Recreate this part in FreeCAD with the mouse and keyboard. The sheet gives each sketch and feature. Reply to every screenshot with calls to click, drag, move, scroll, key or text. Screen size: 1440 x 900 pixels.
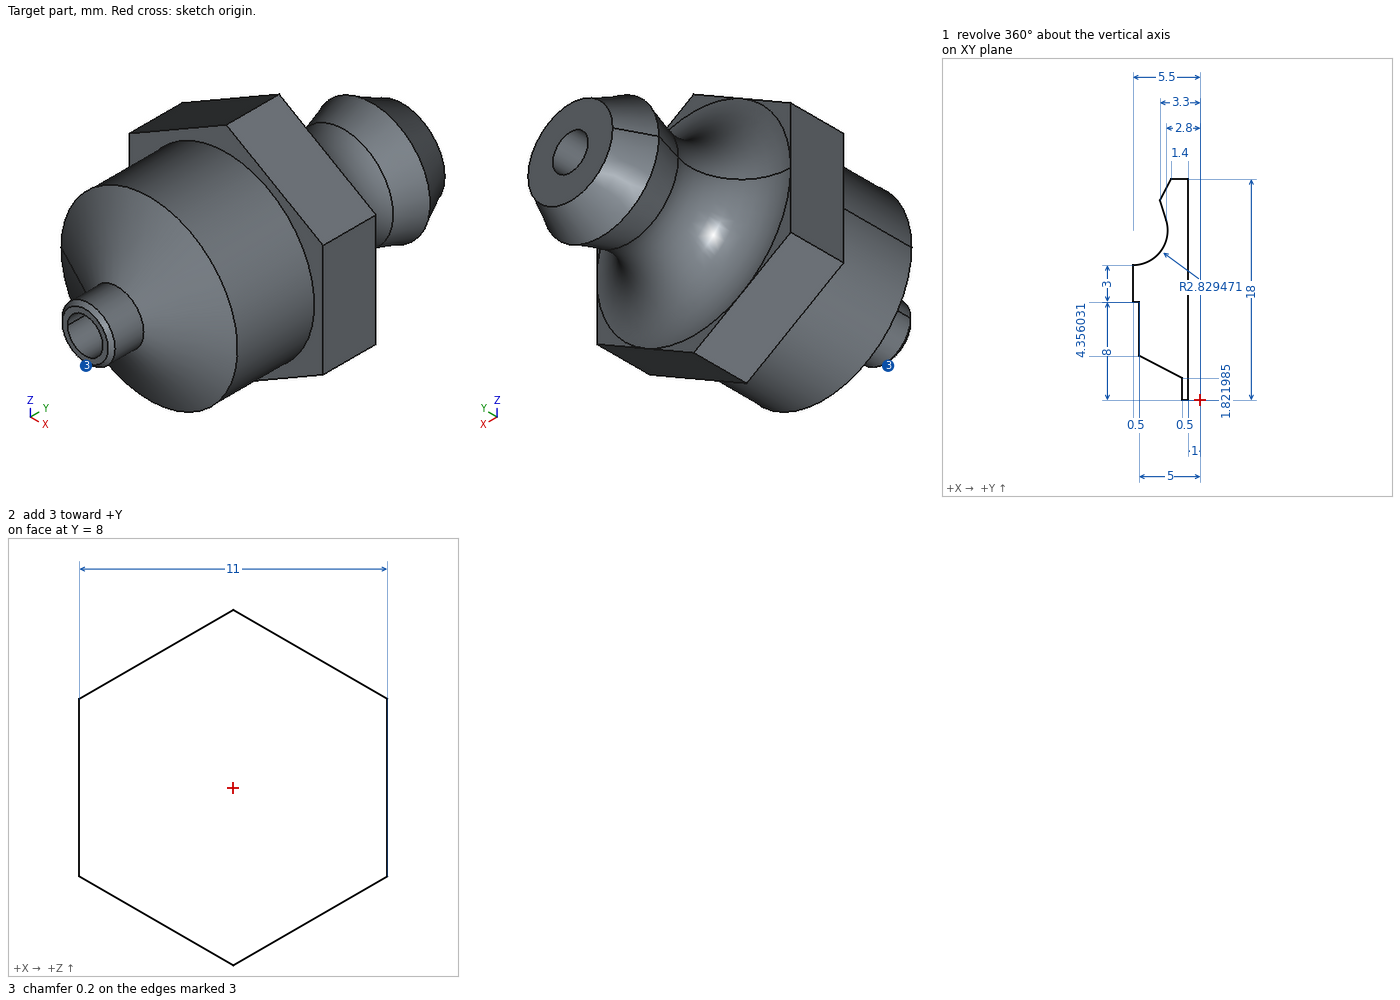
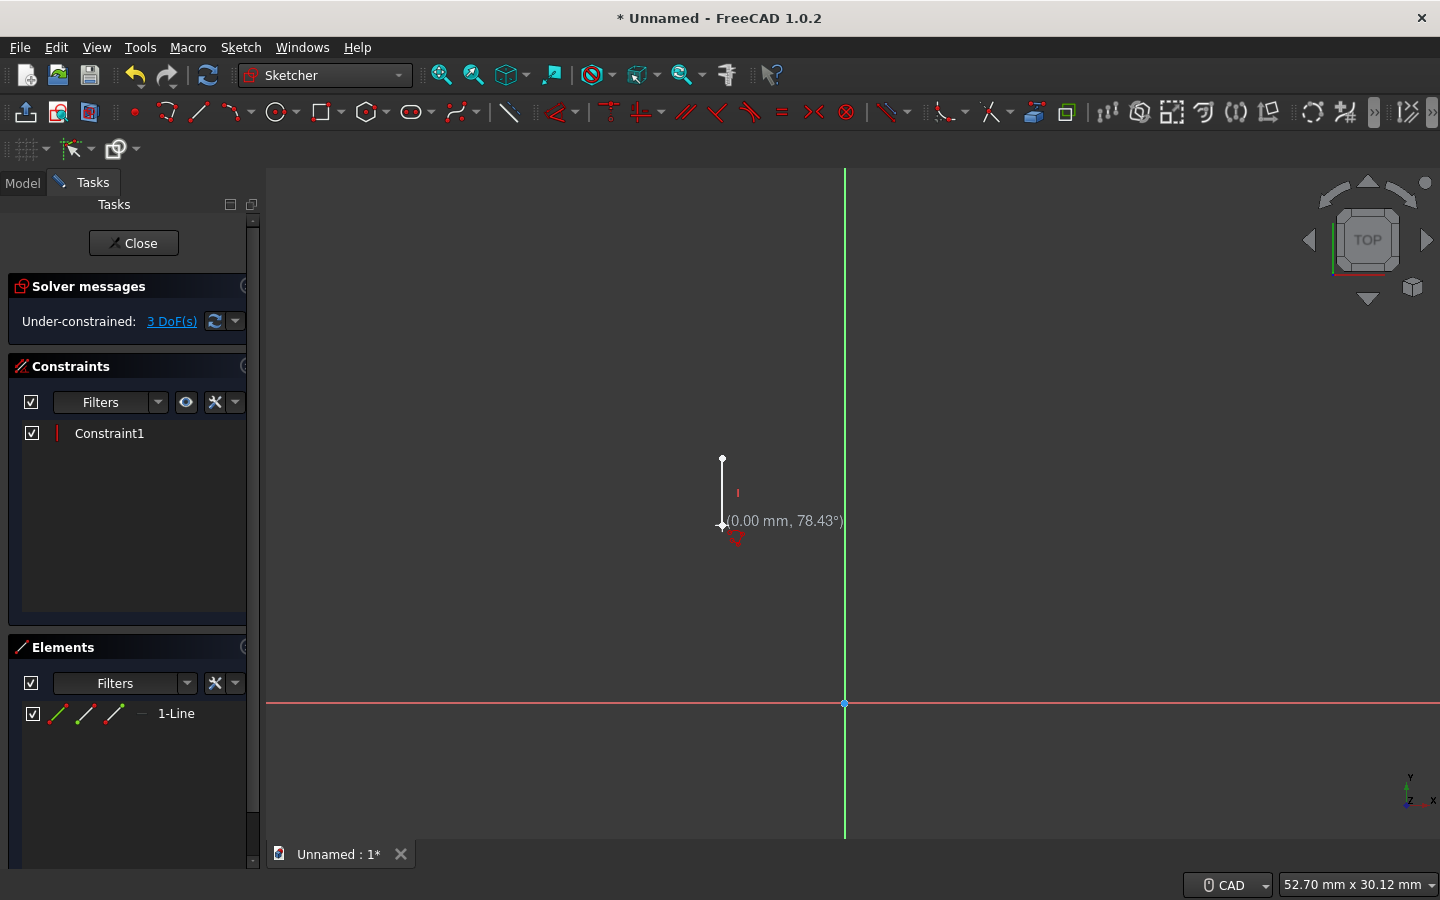
scroll(733, 525, up, 2)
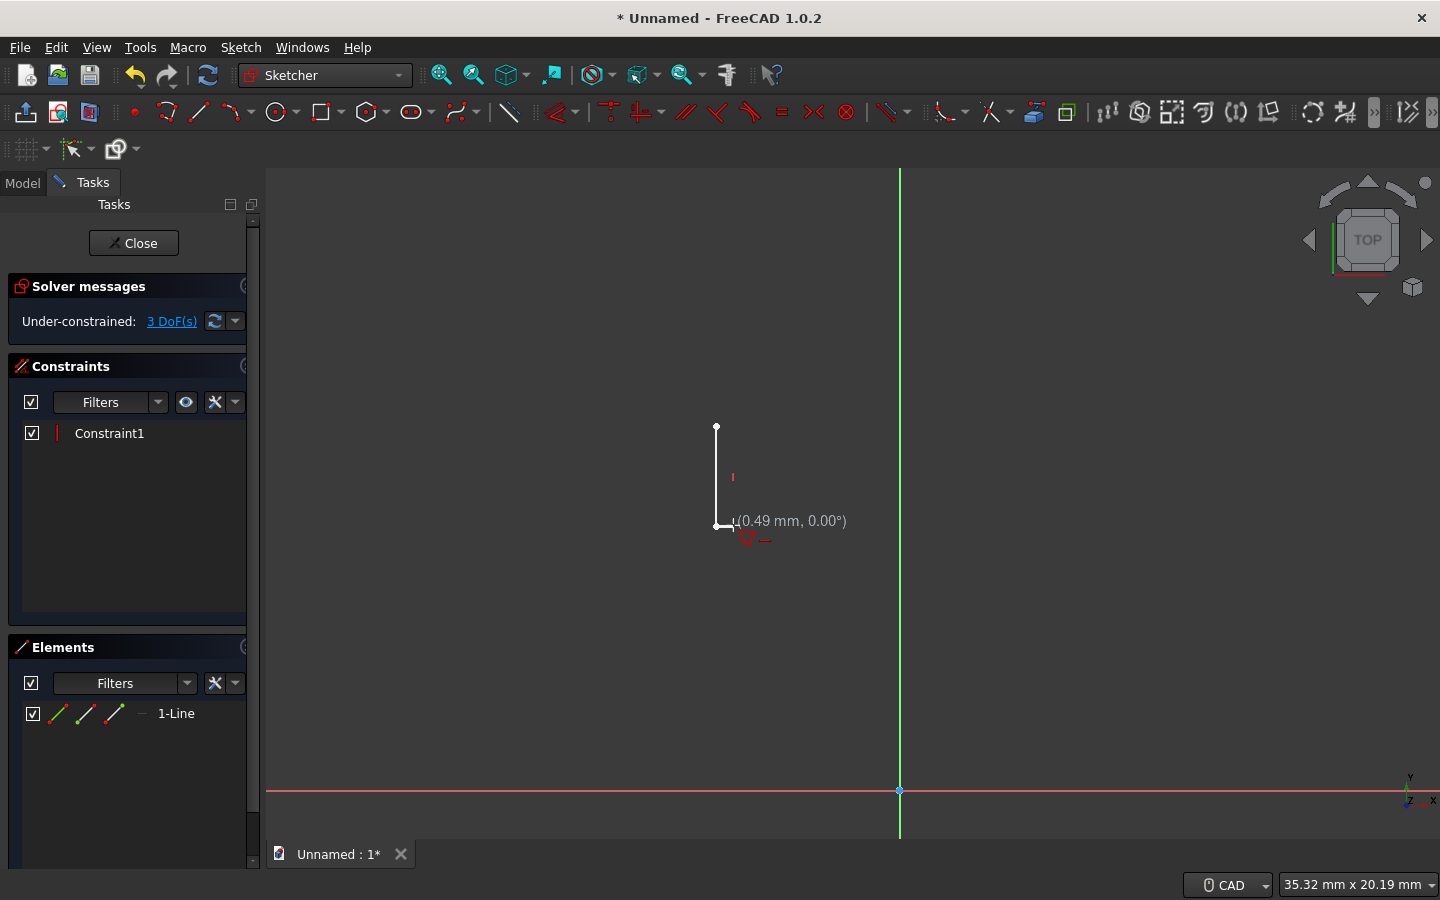
click(734, 525)
click(734, 670)
click(850, 730)
click(850, 791)
click(866, 782)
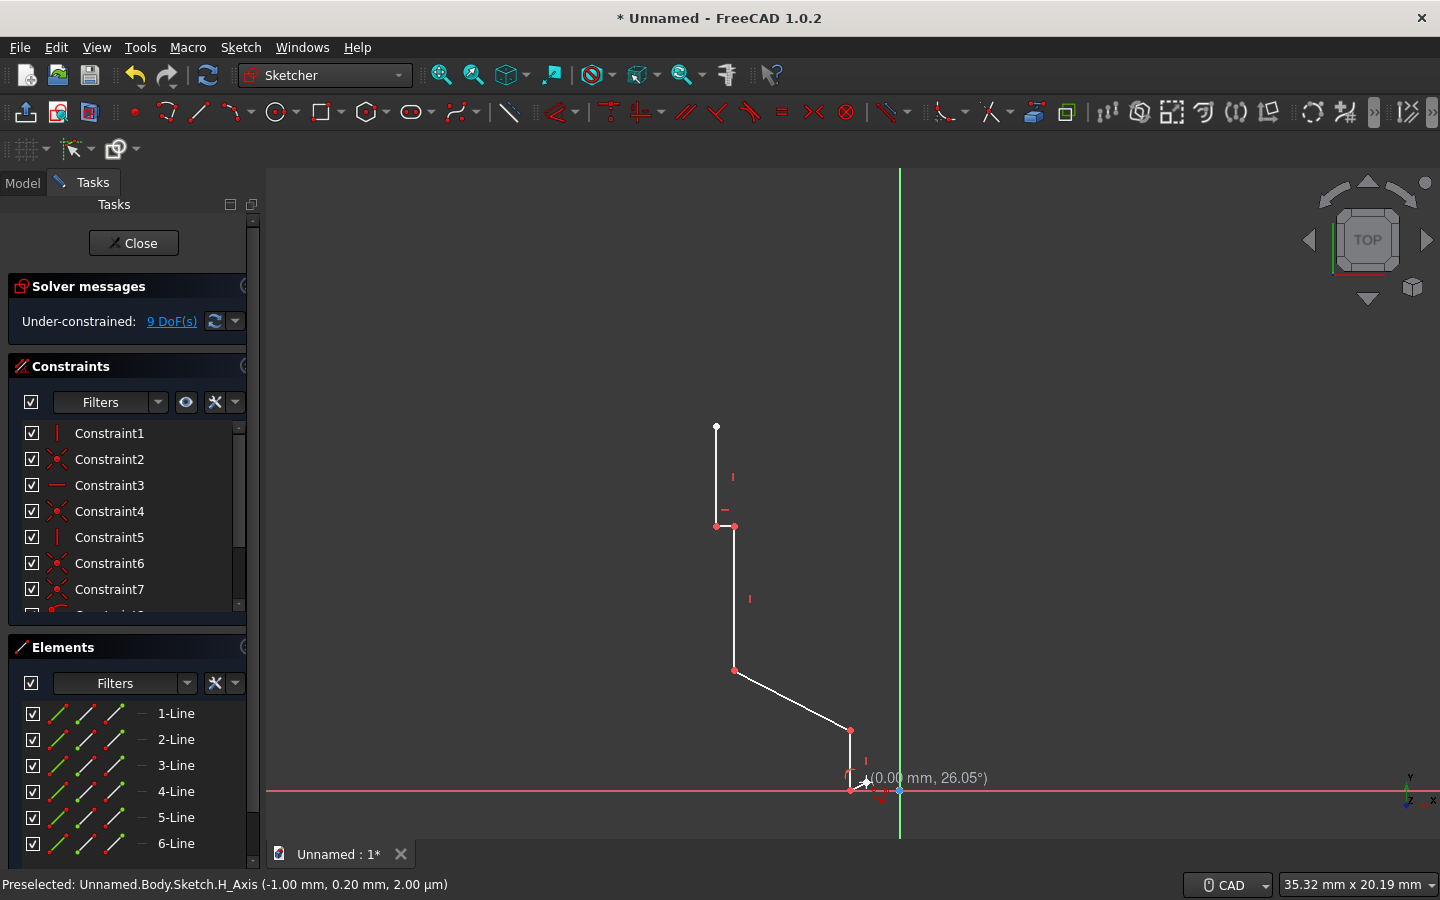
scroll(736, 528, down, 2)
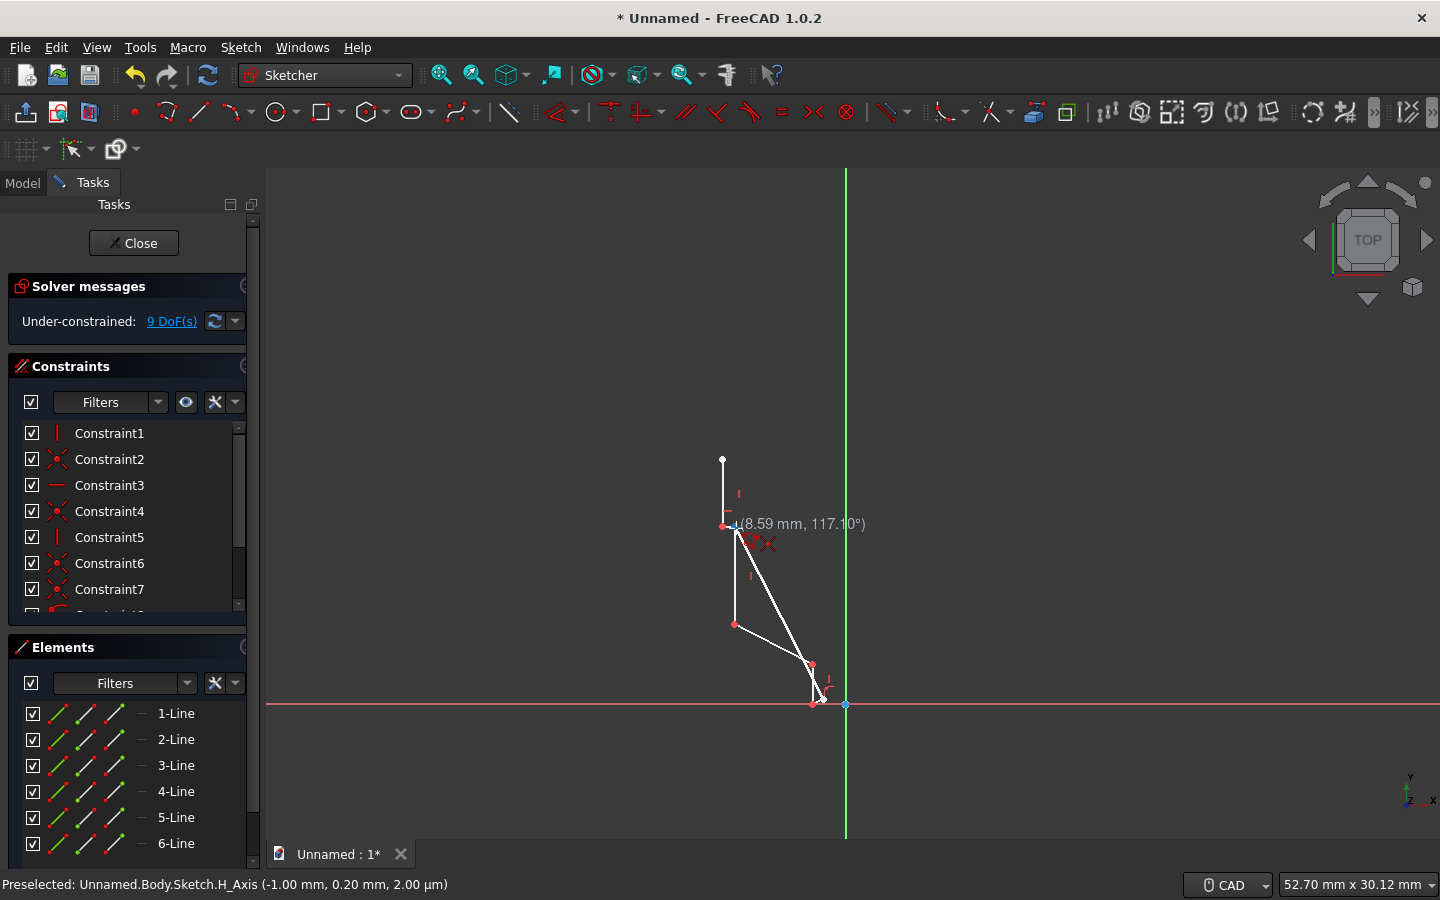
click(823, 303)
click(792, 303)
click(772, 342)
click(783, 377)
right_click(783, 377)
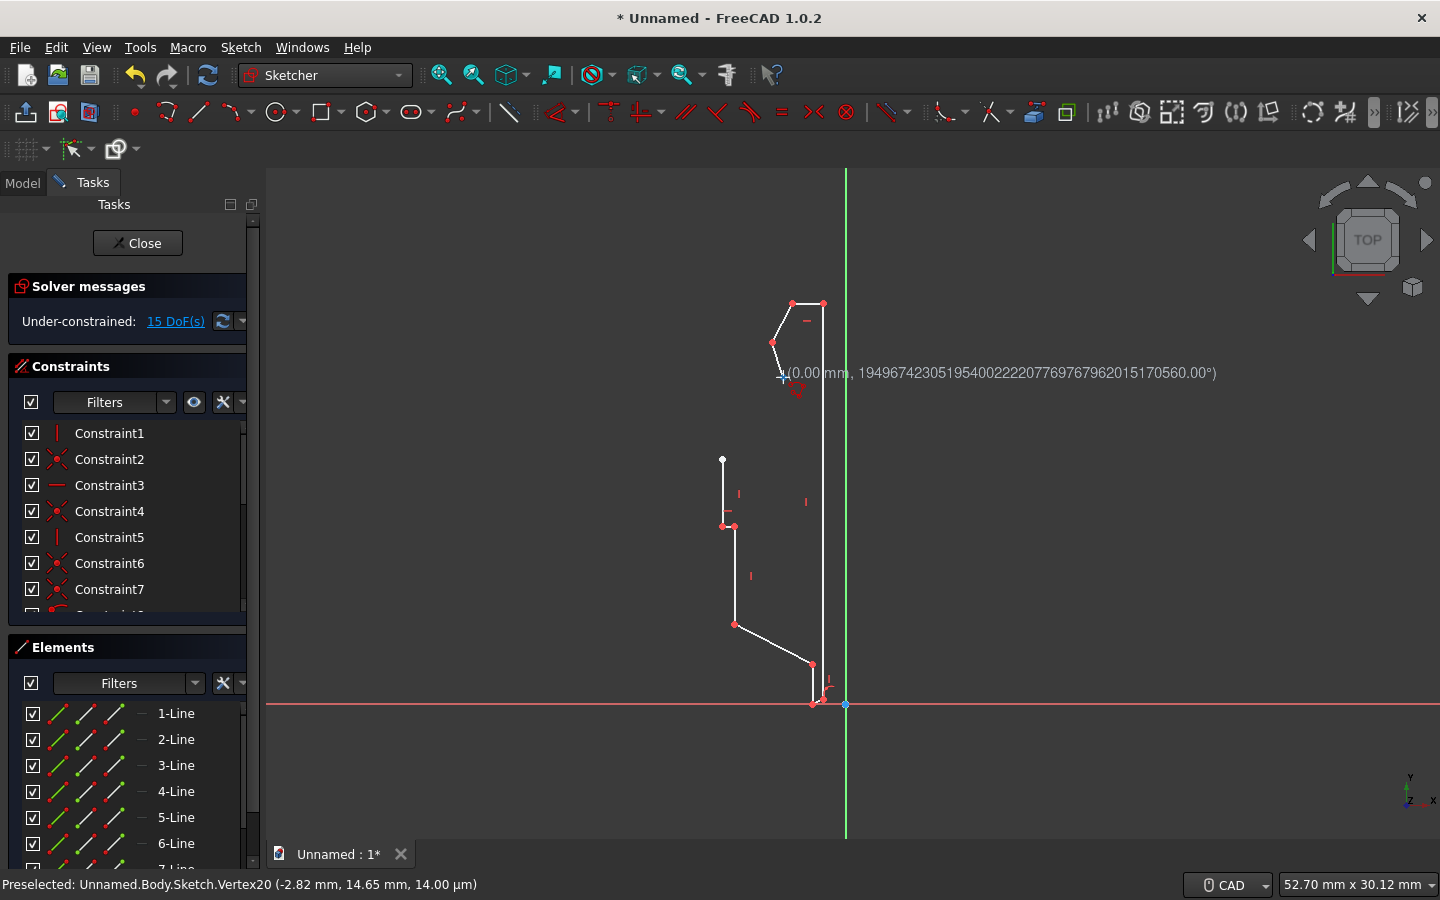
click(232, 112)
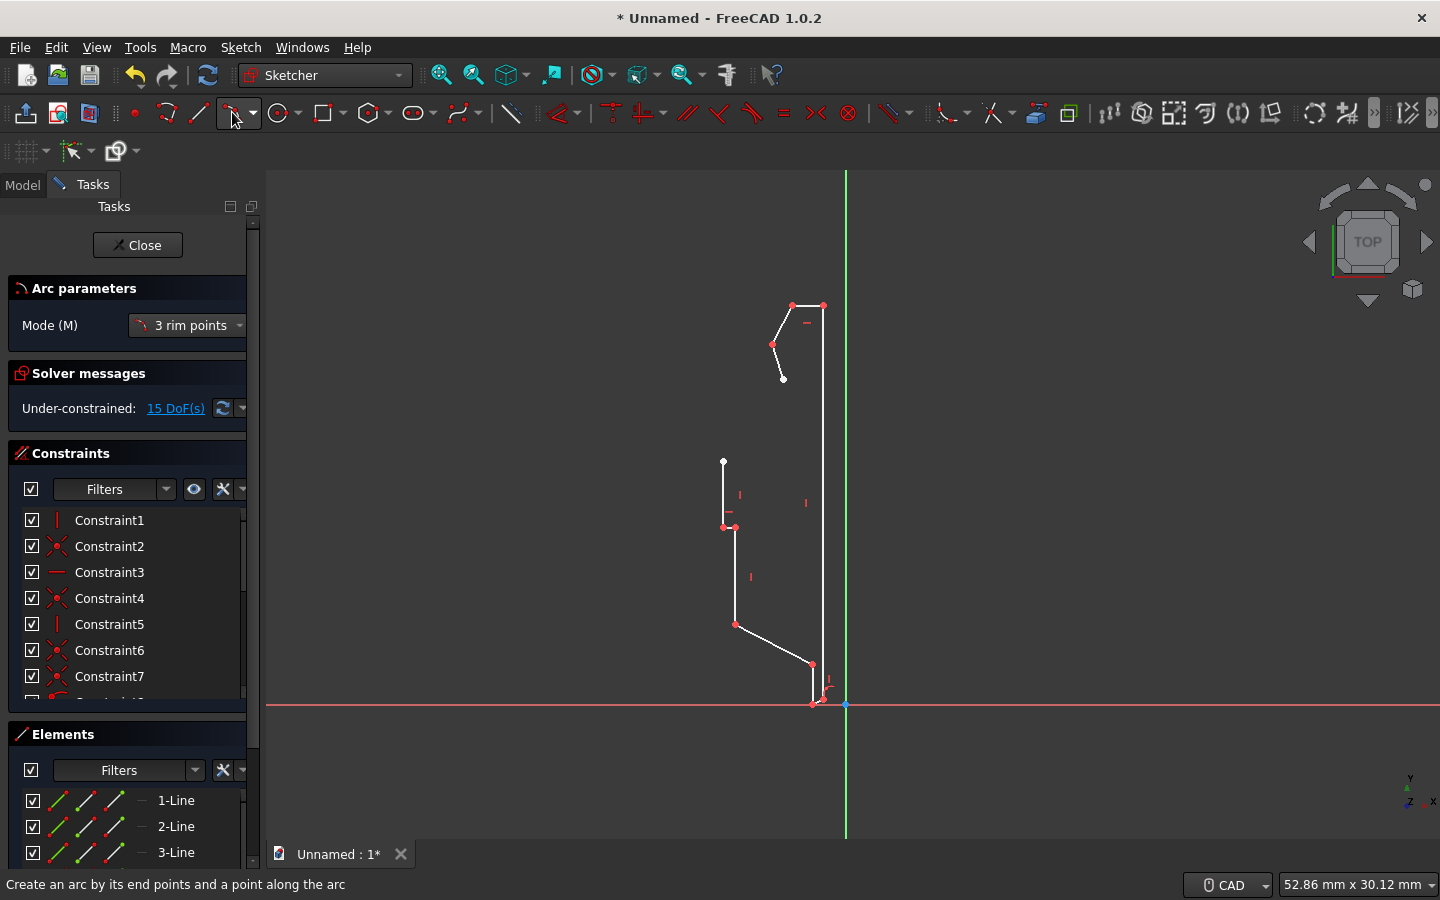
click(783, 379)
click(723, 461)
click(774, 435)
key(Escape)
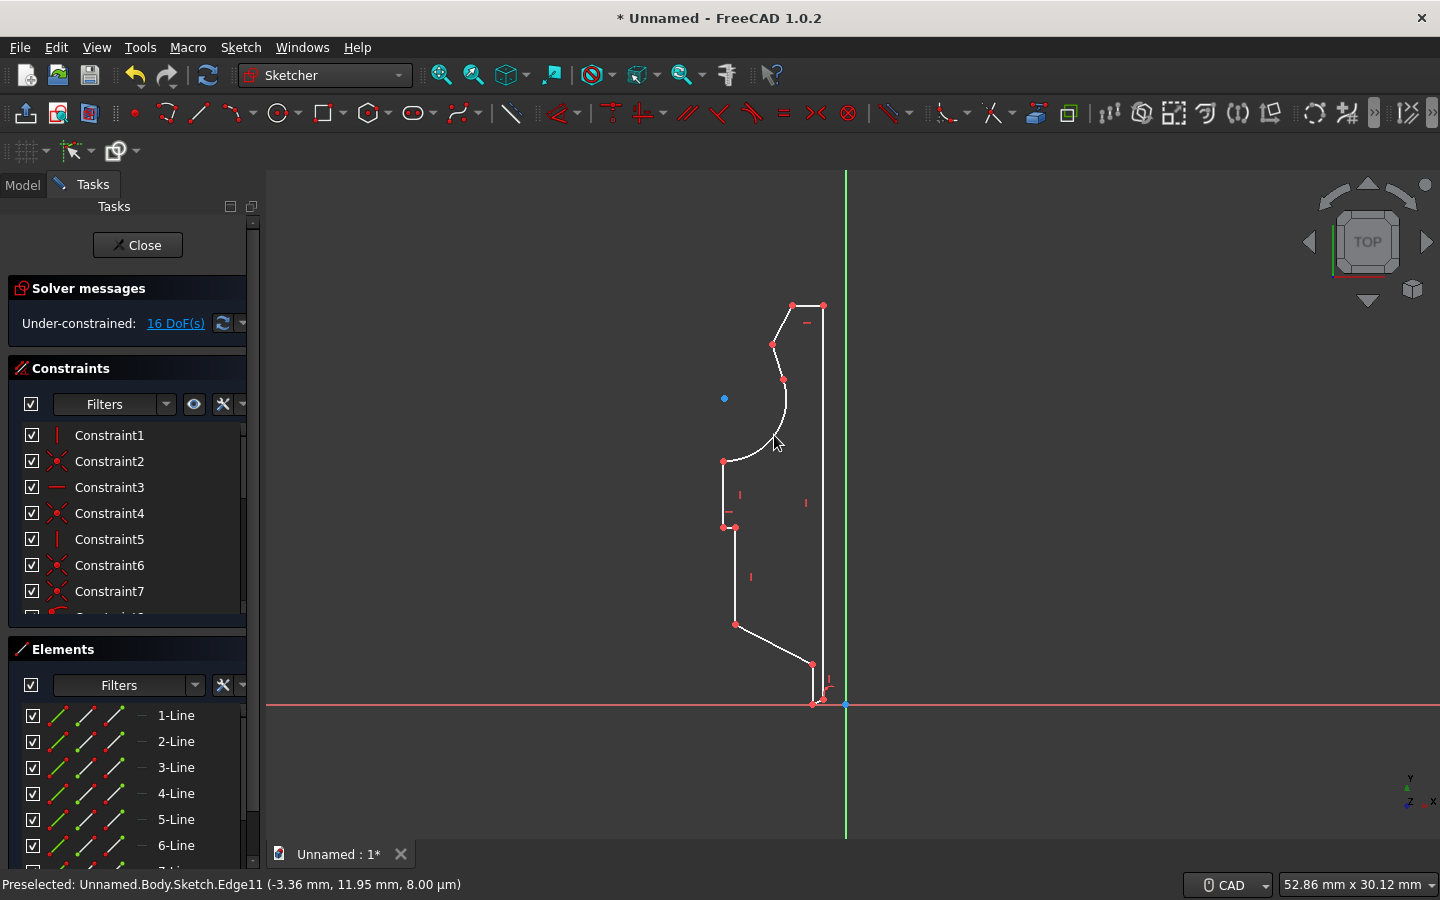
scroll(776, 355, up, 2)